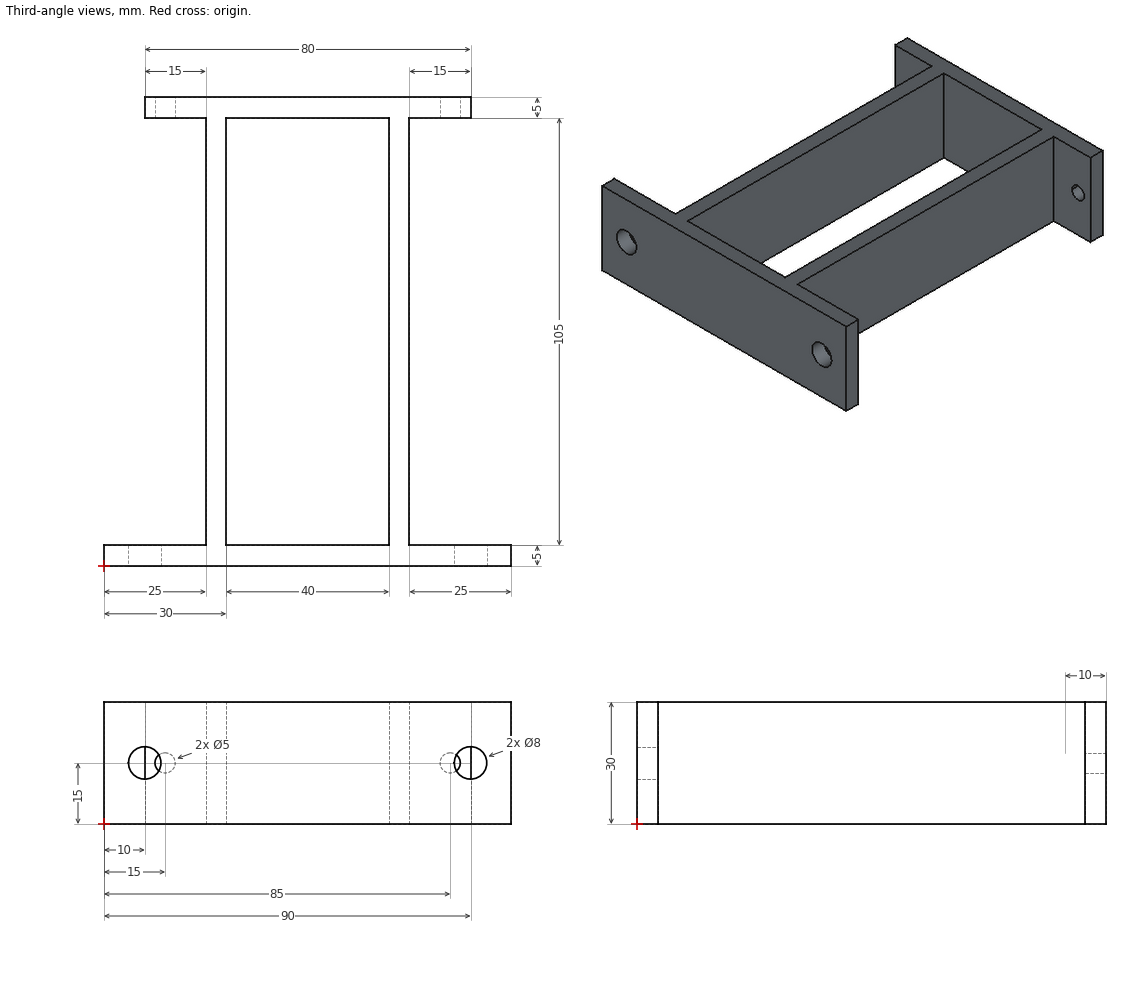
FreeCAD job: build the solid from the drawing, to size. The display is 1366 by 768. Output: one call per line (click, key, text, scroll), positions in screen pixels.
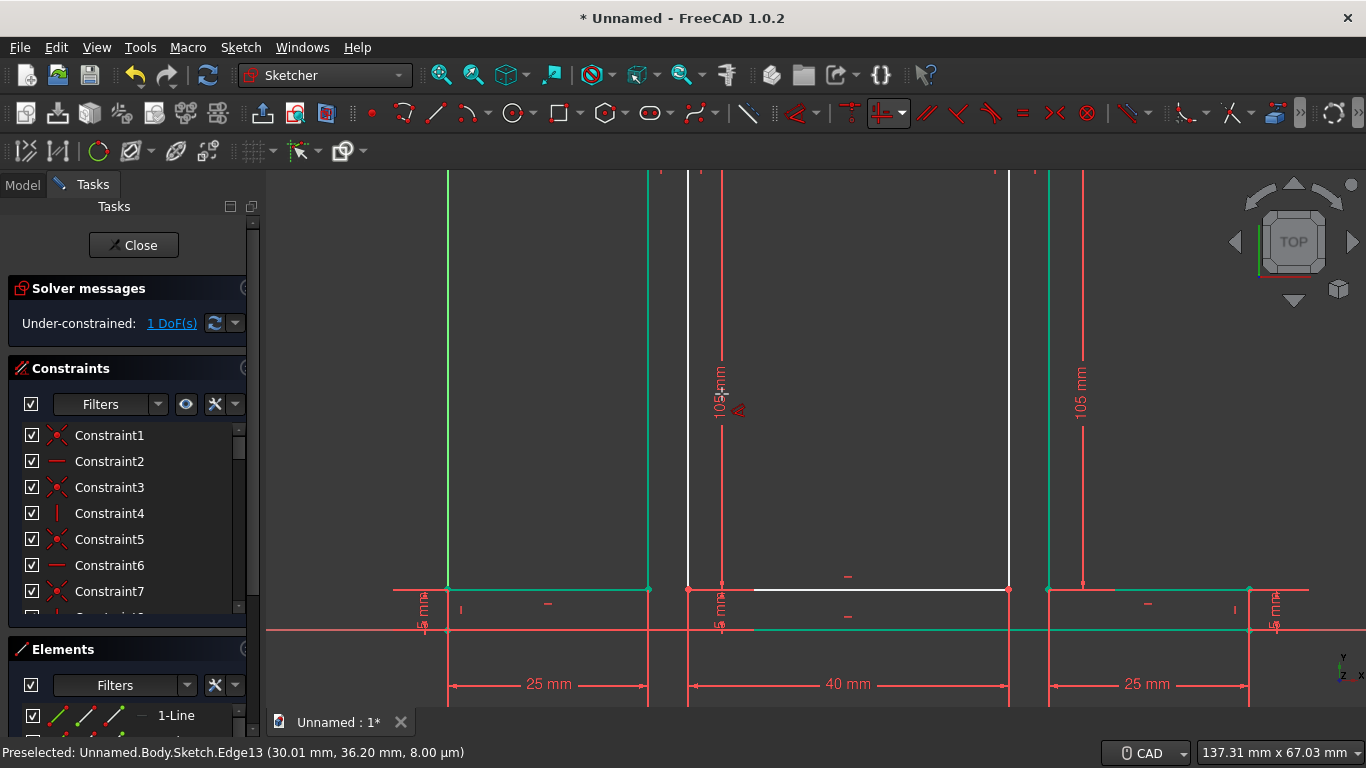
scroll(689, 595, down, 5)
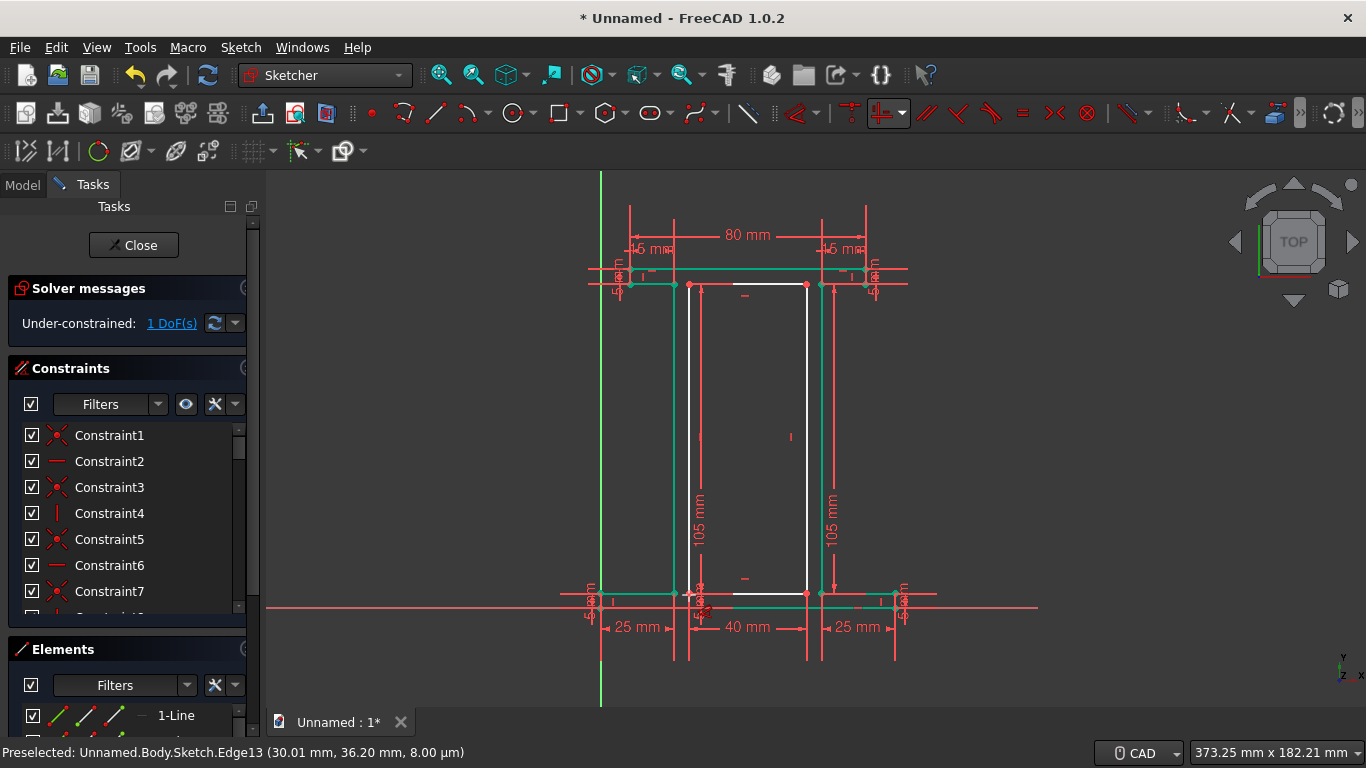
click(689, 284)
click(645, 666)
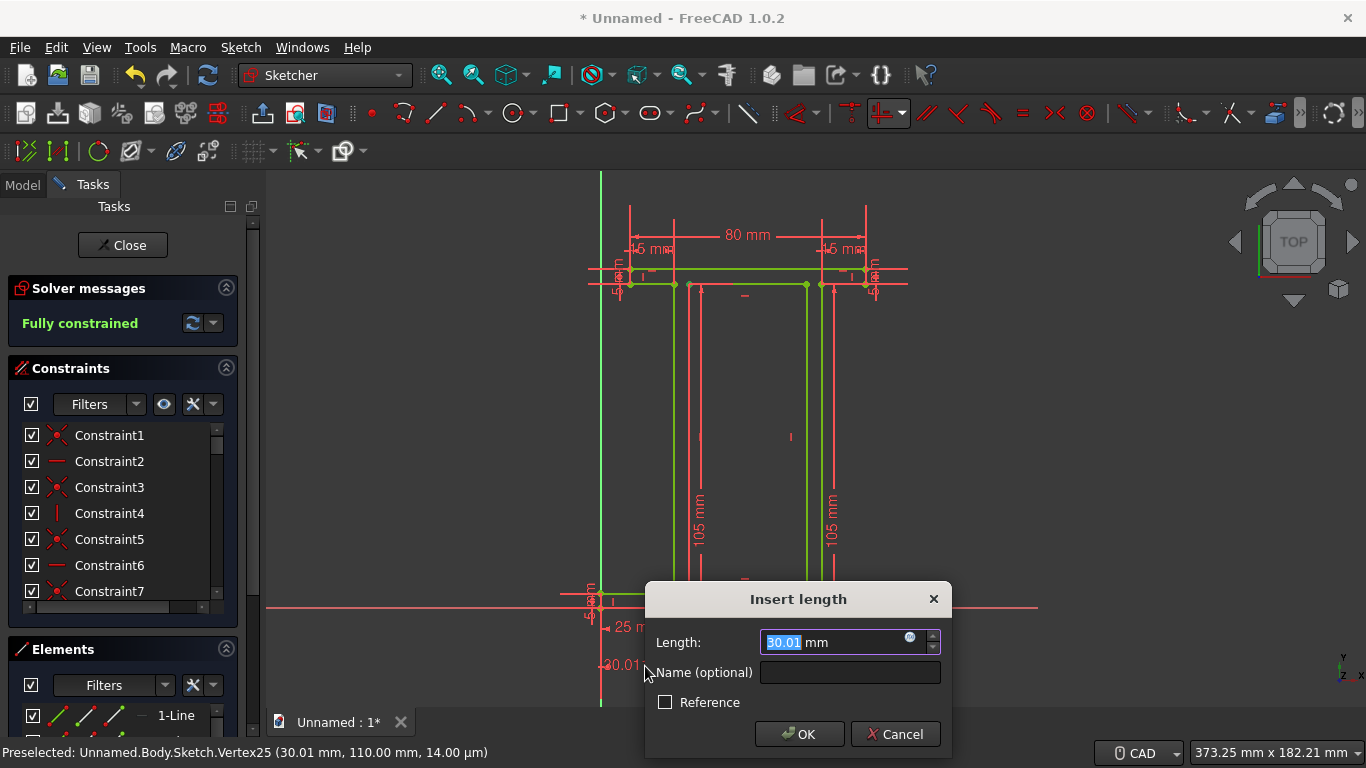
text(30)
key(Return)
key(Escape)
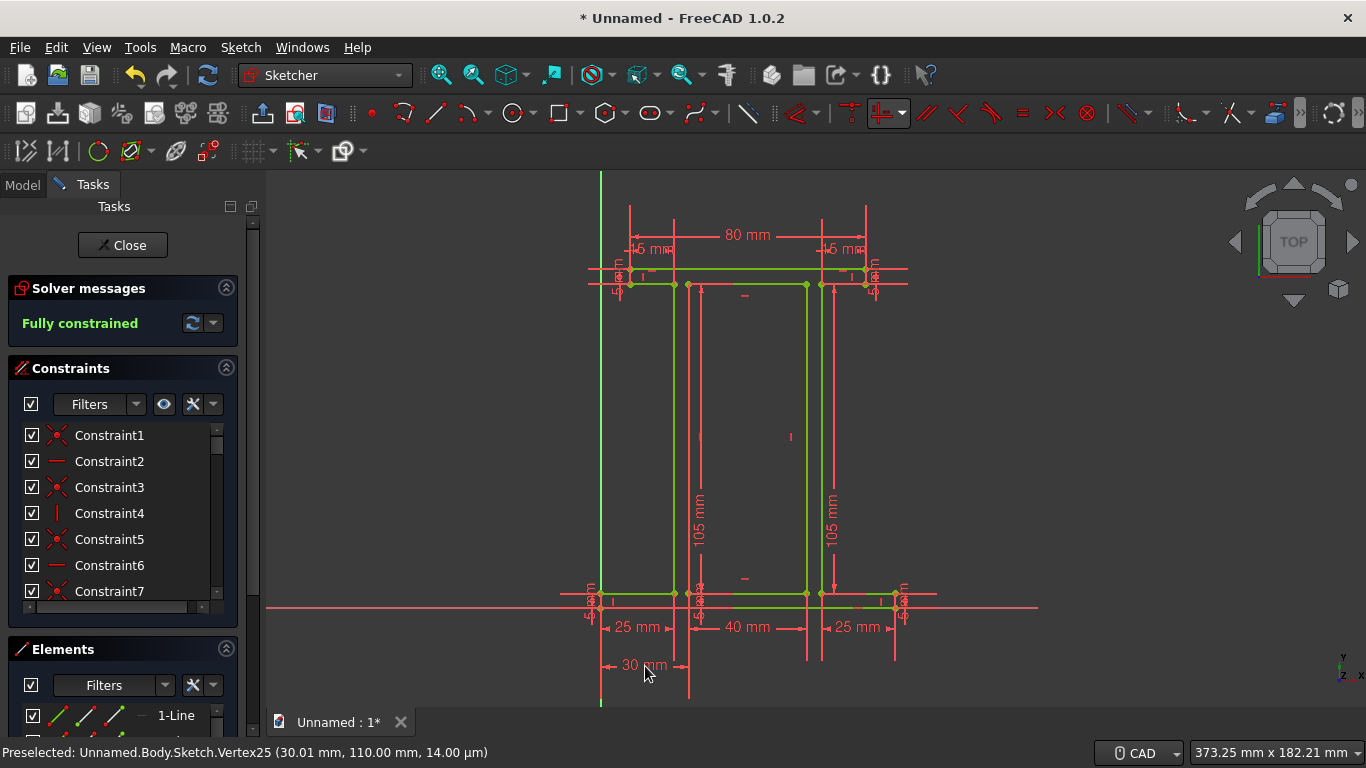
click(123, 245)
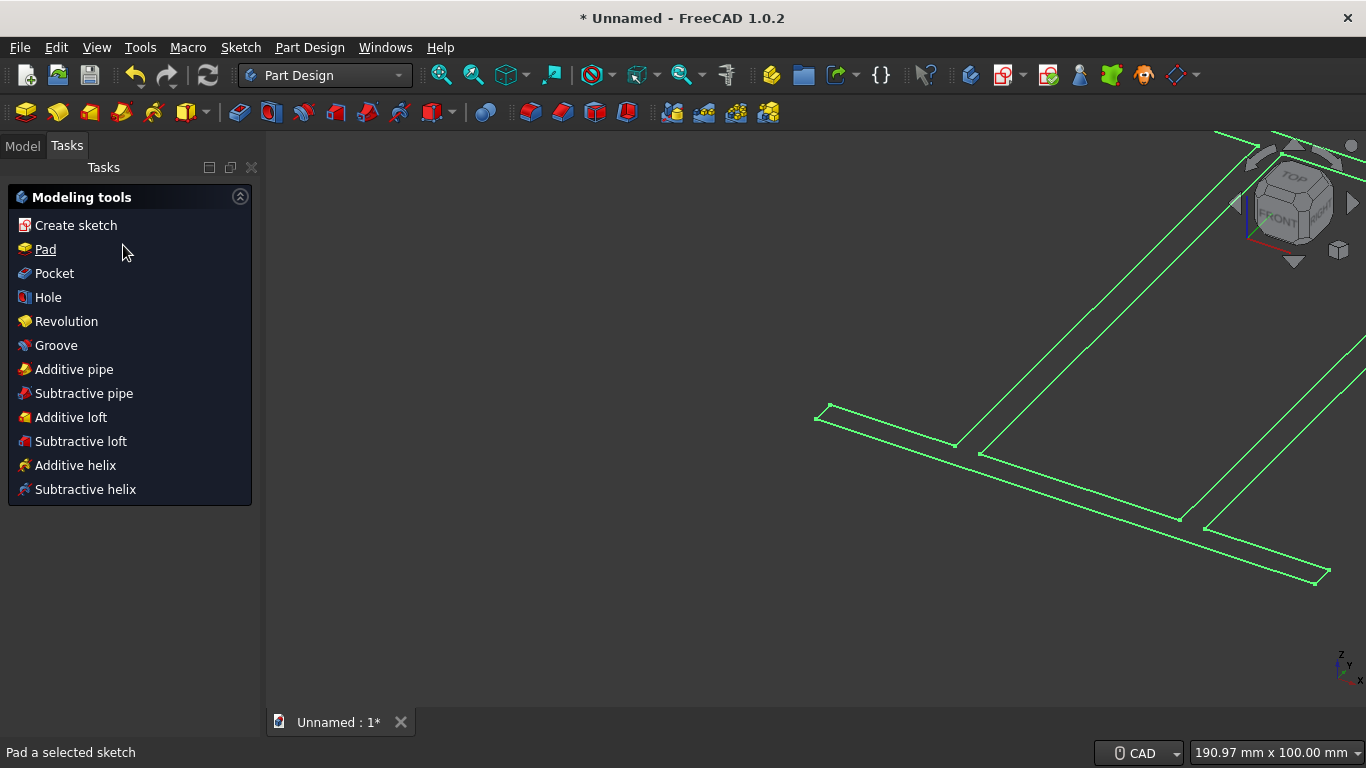
click(26, 112)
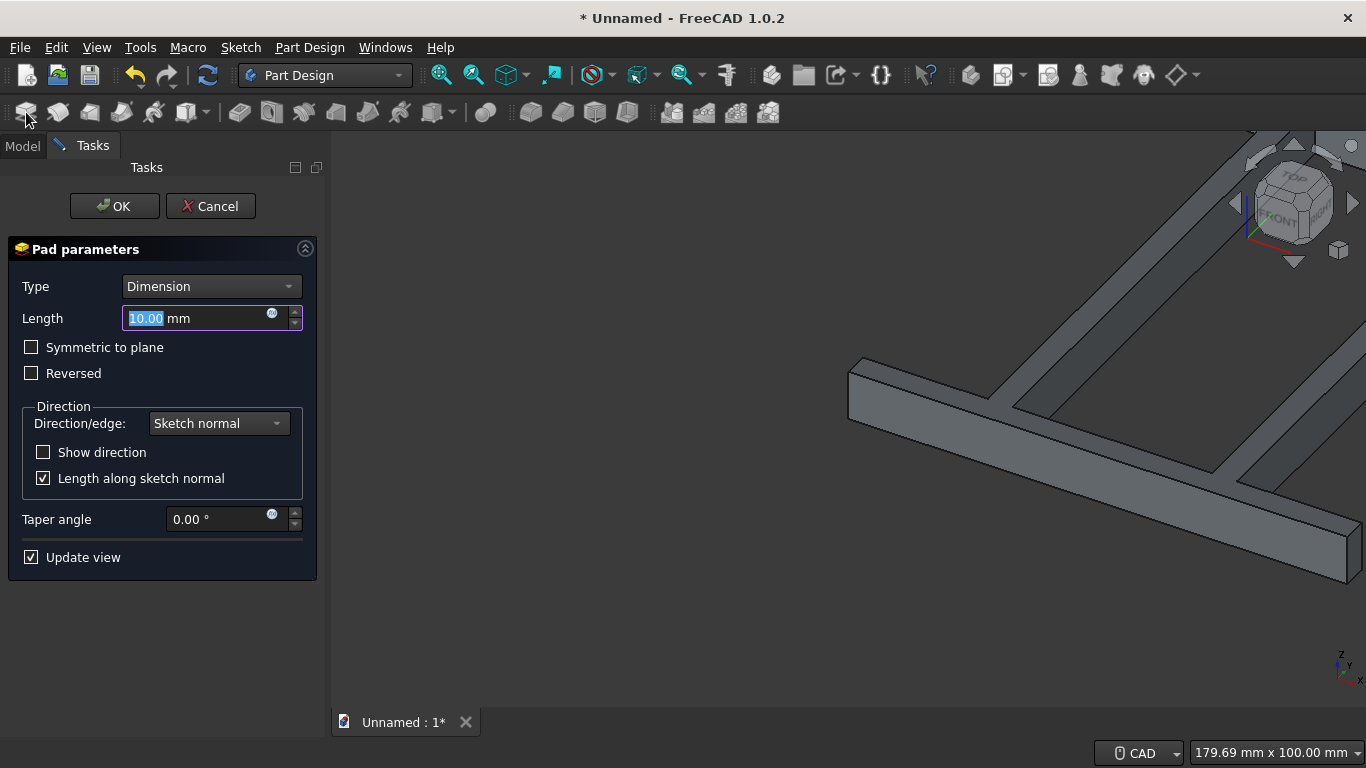
text(30)
key(Tab)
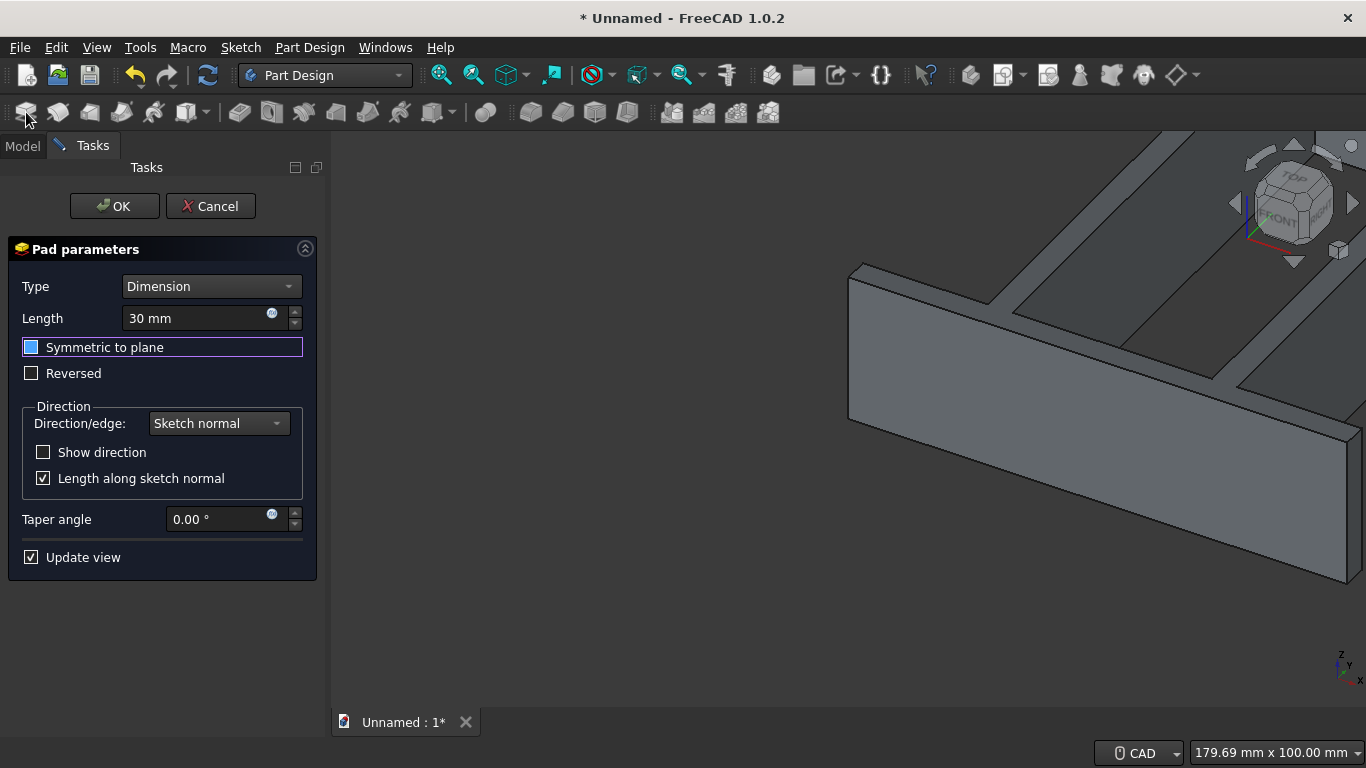
click(115, 206)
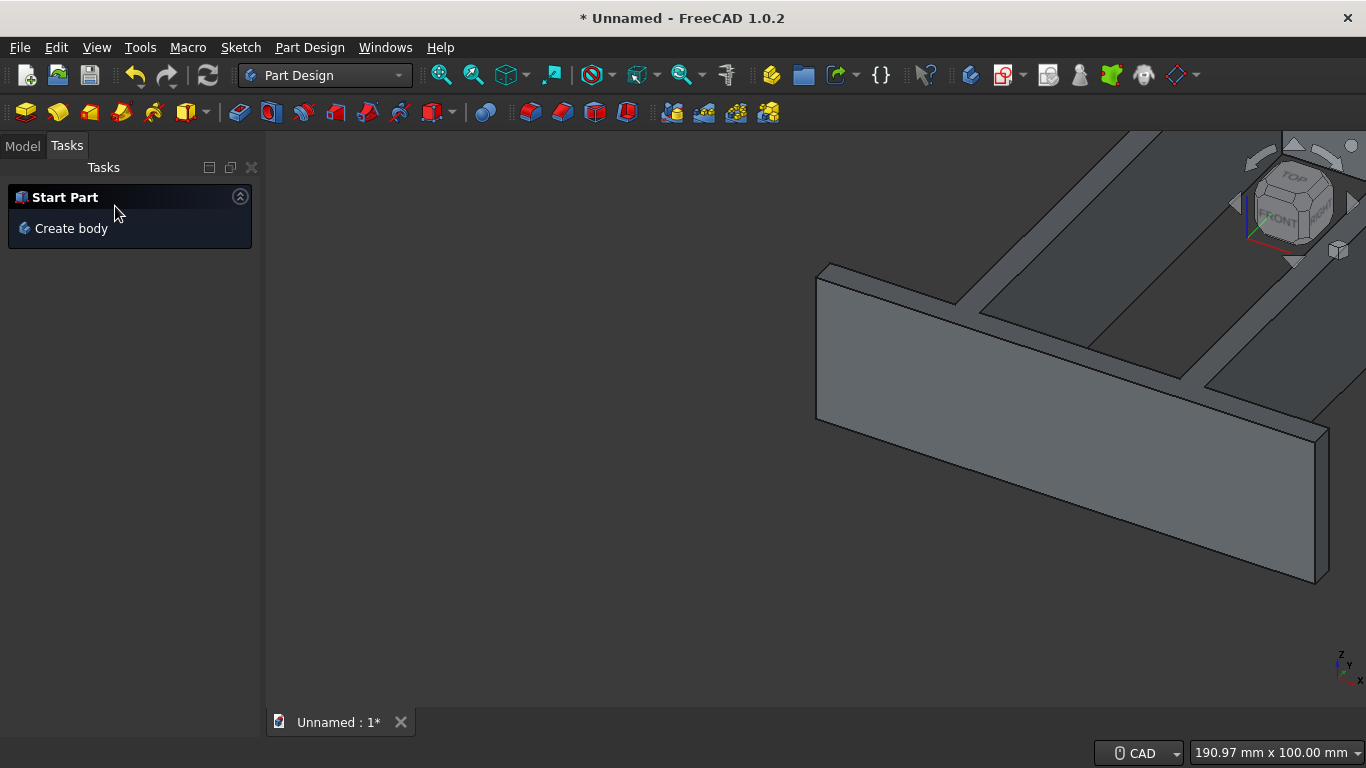
click(442, 76)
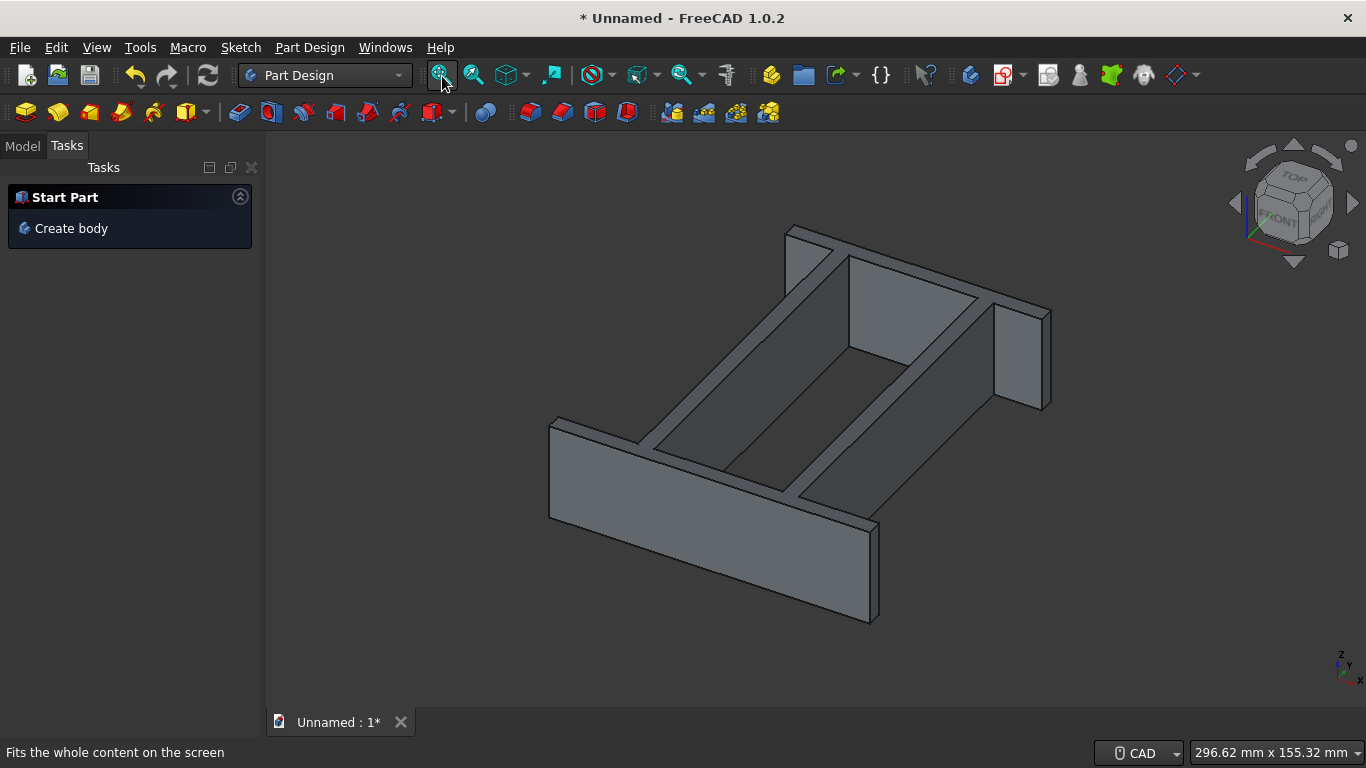
key(4)